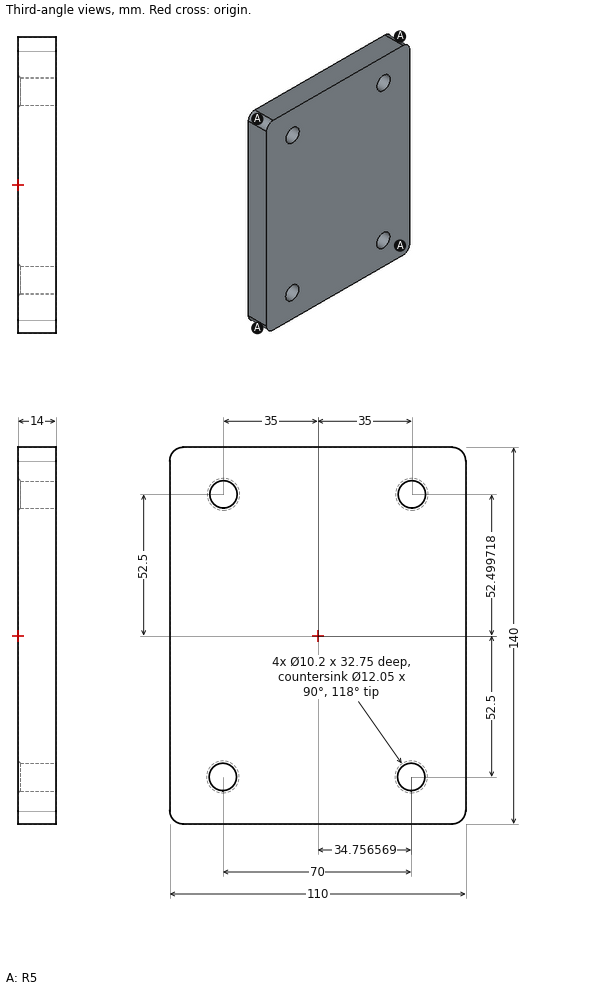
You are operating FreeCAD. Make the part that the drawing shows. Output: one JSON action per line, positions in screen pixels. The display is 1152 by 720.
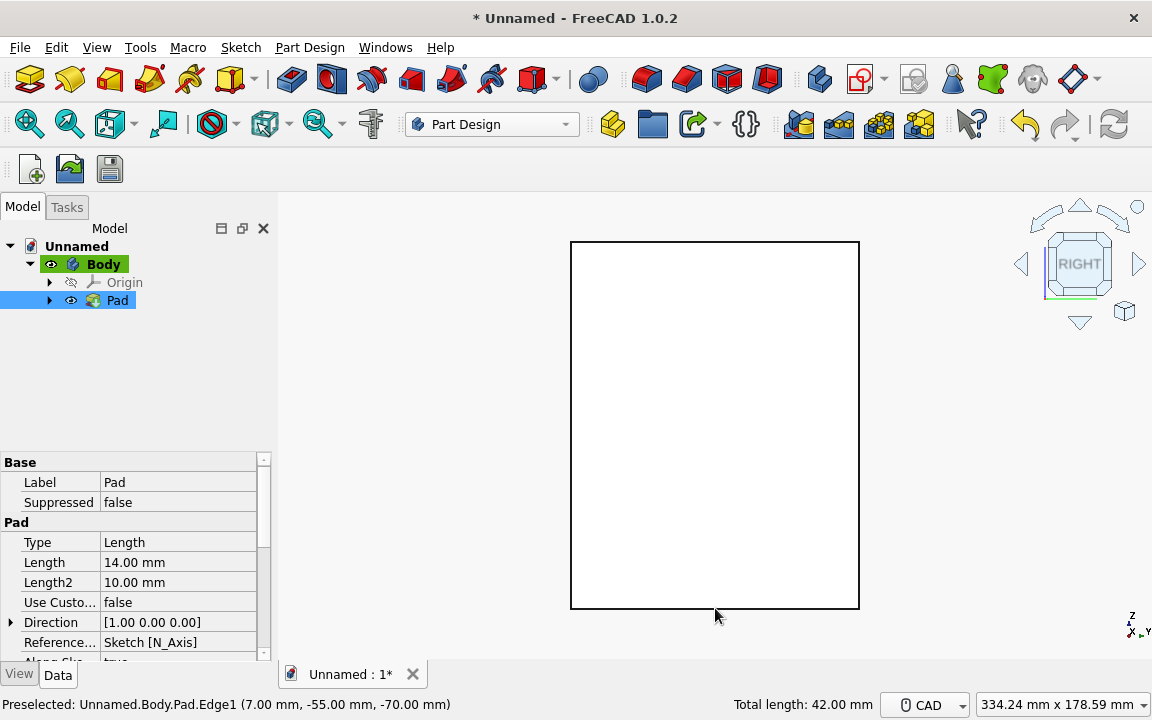
{"action": "key", "text": "5"}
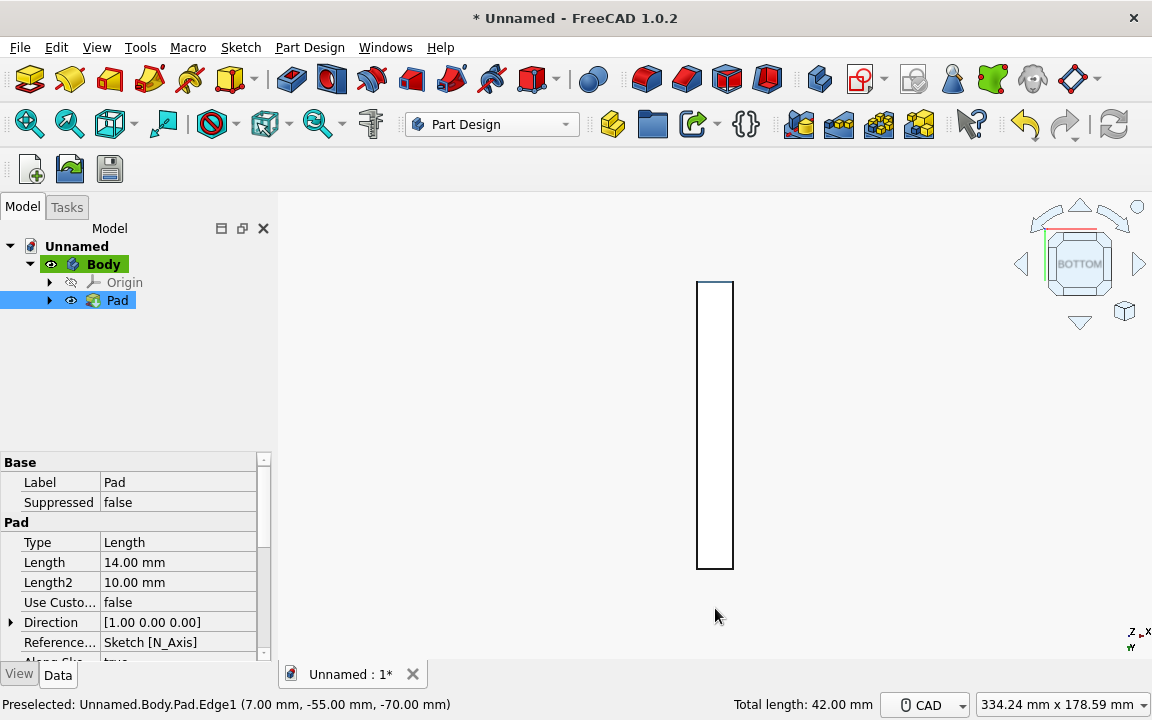
{"action": "left_click", "coordinate": [715, 568], "text": "ctrl"}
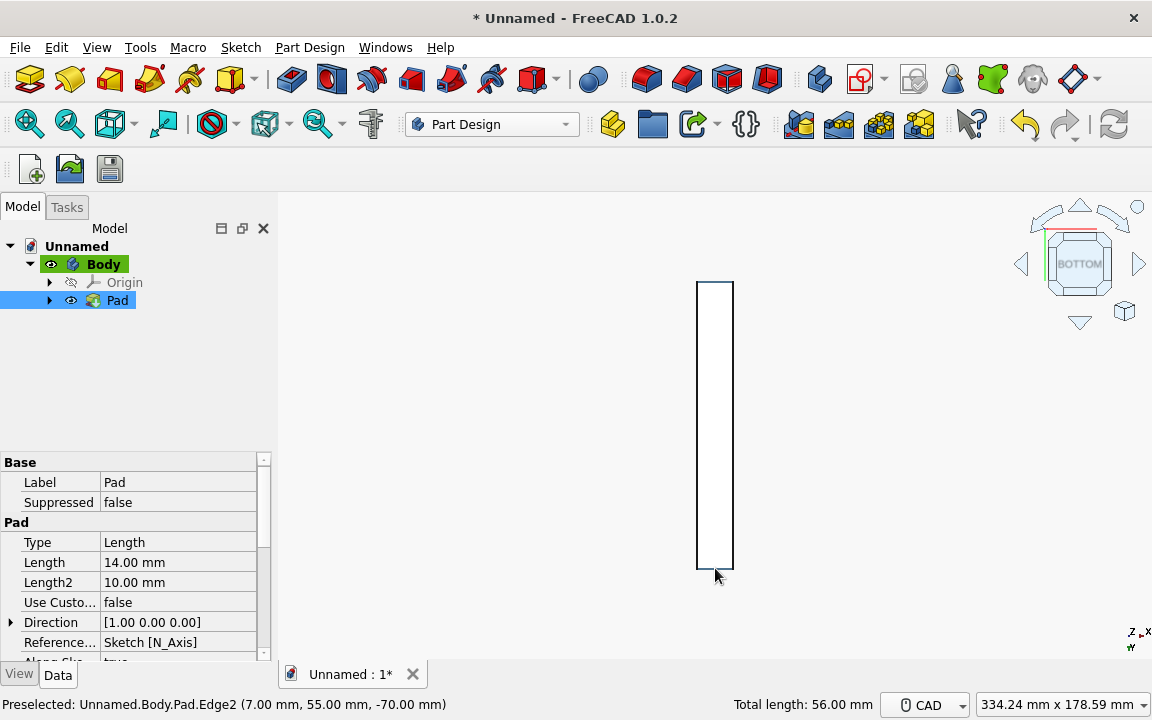
{"action": "left_click", "coordinate": [648, 80]}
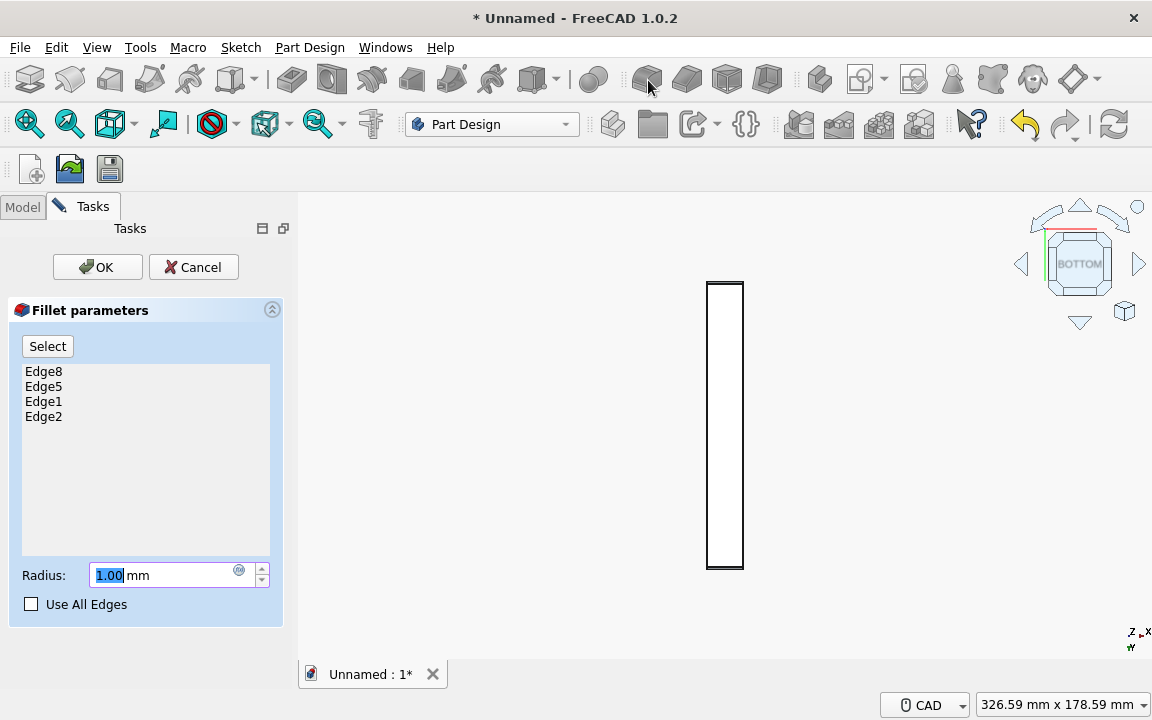
{"action": "type", "text": "5"}
{"action": "key", "text": "Tab"}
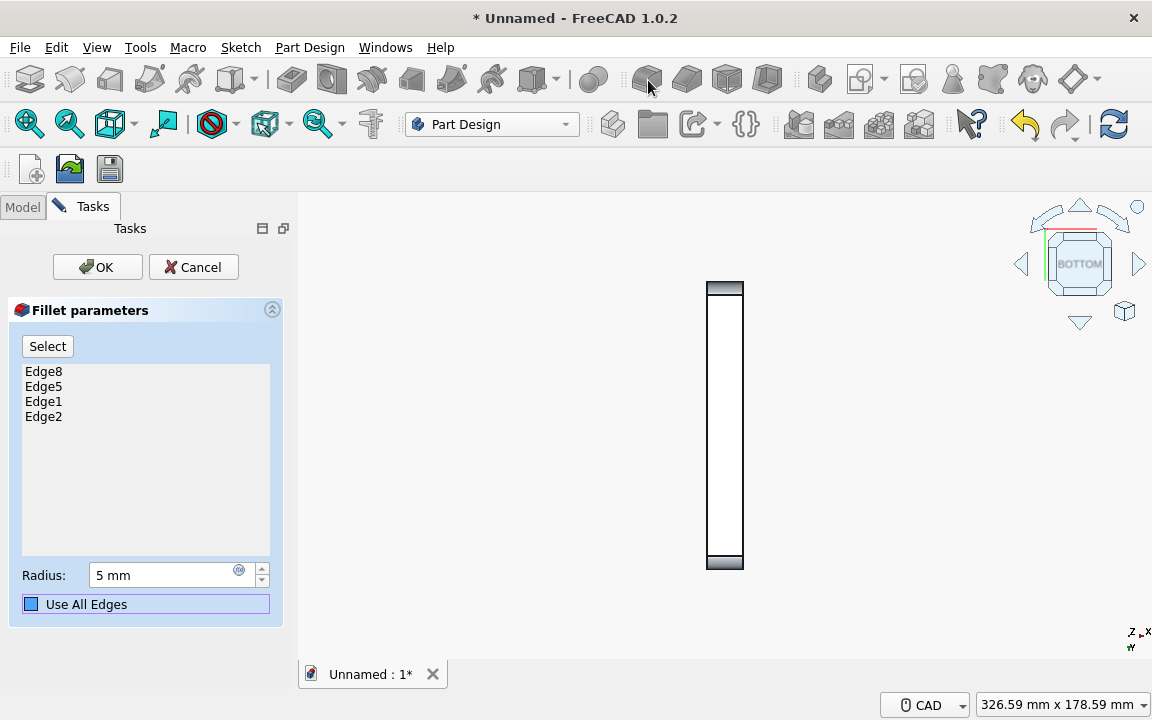
{"action": "left_click", "coordinate": [98, 267]}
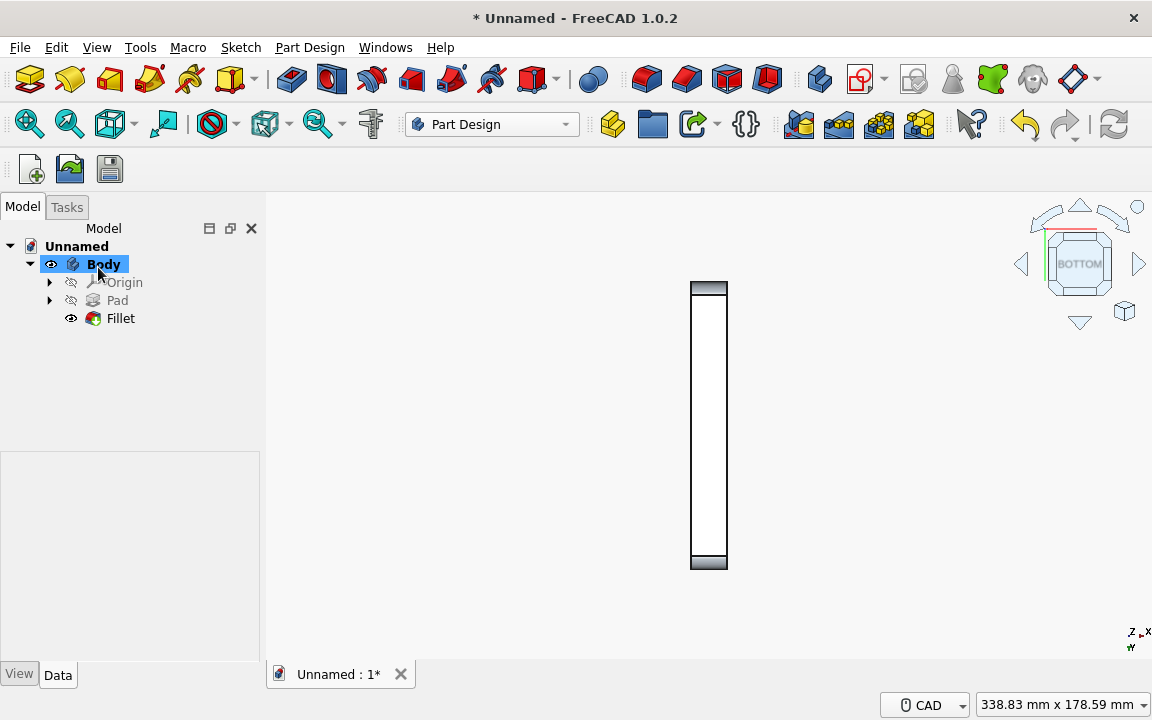
{"action": "key", "text": "6"}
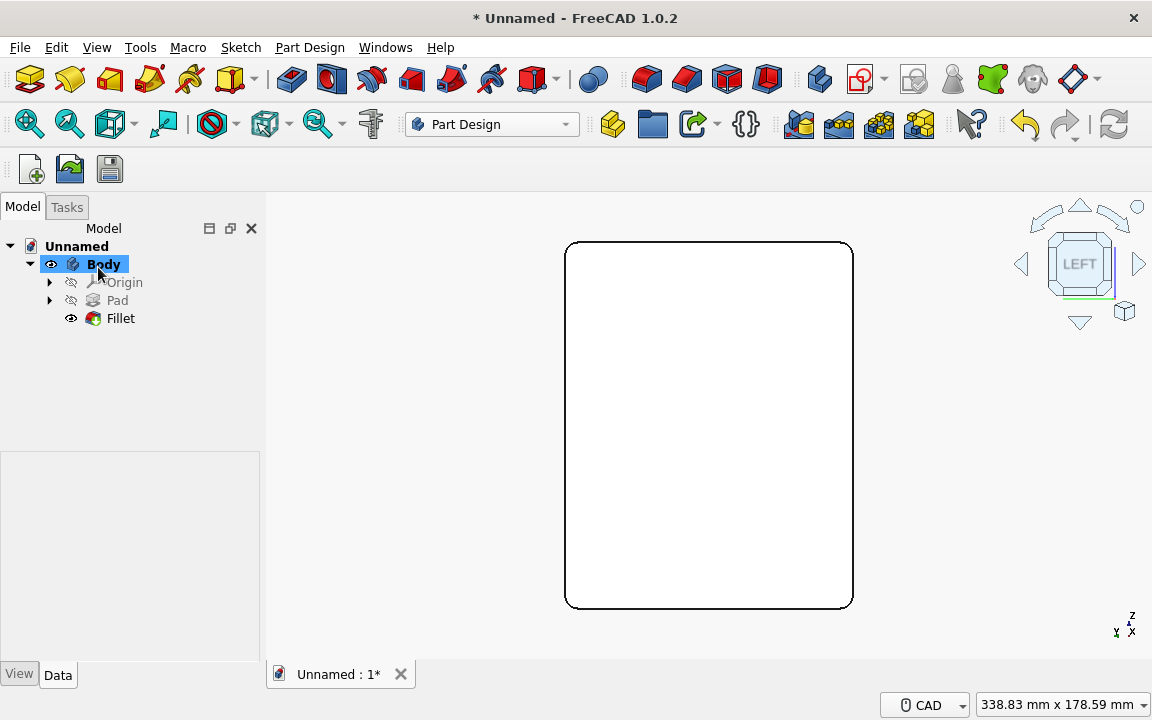
{"action": "left_click", "coordinate": [709, 424]}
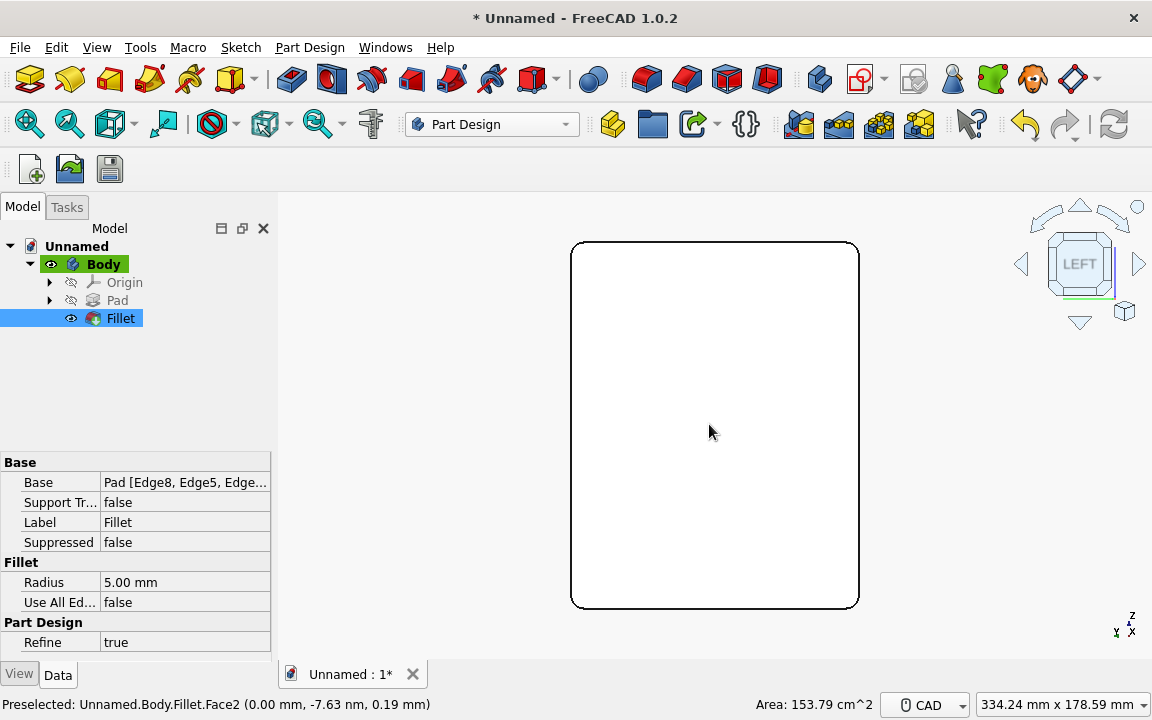
{"action": "left_click", "coordinate": [860, 80]}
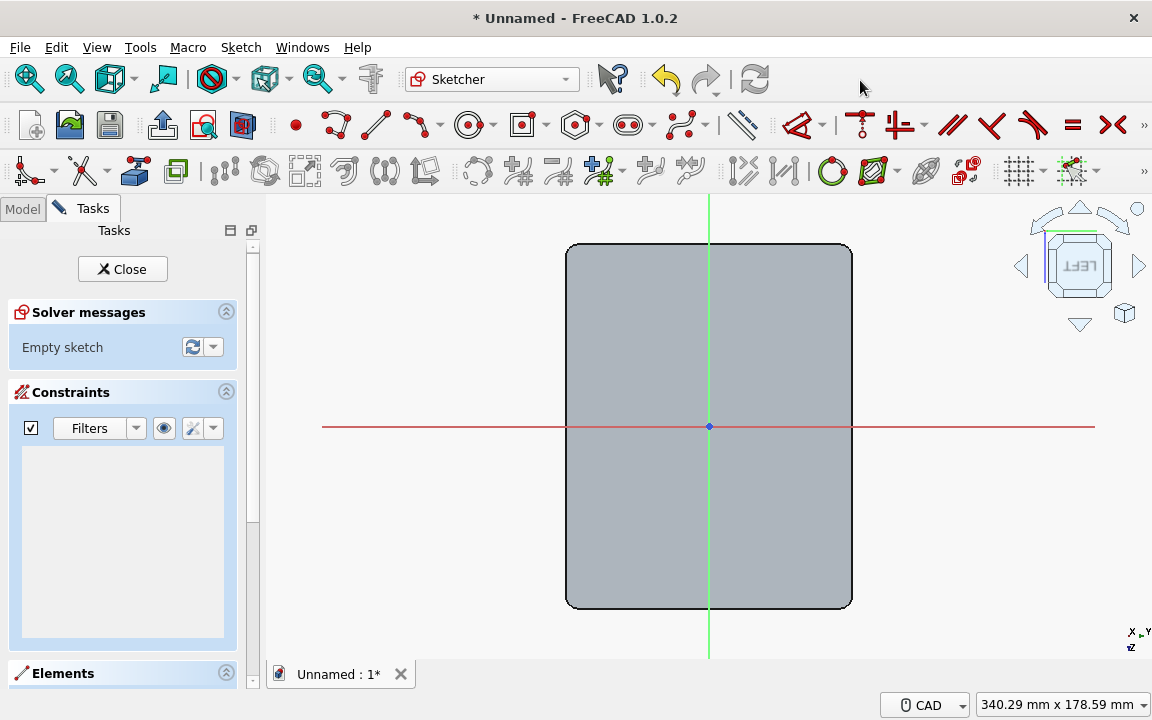
{"action": "left_click", "coordinate": [470, 126]}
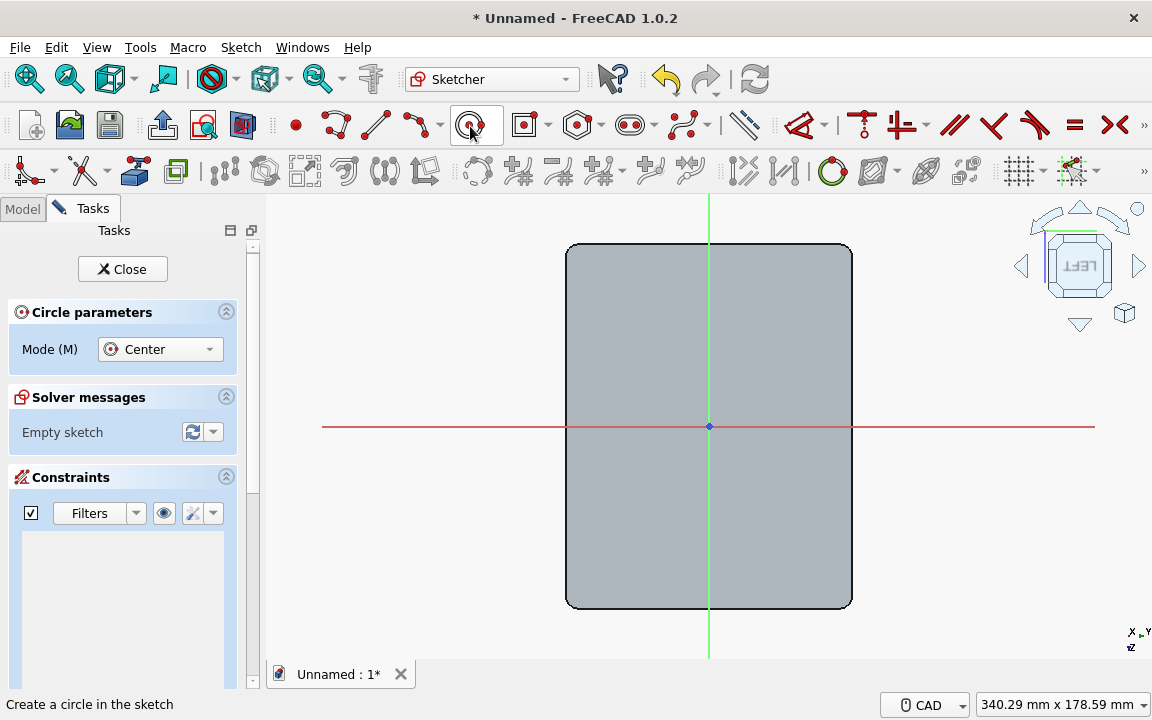
{"action": "scroll", "coordinate": [799, 290], "scroll_direction": "up", "scroll_amount": 3}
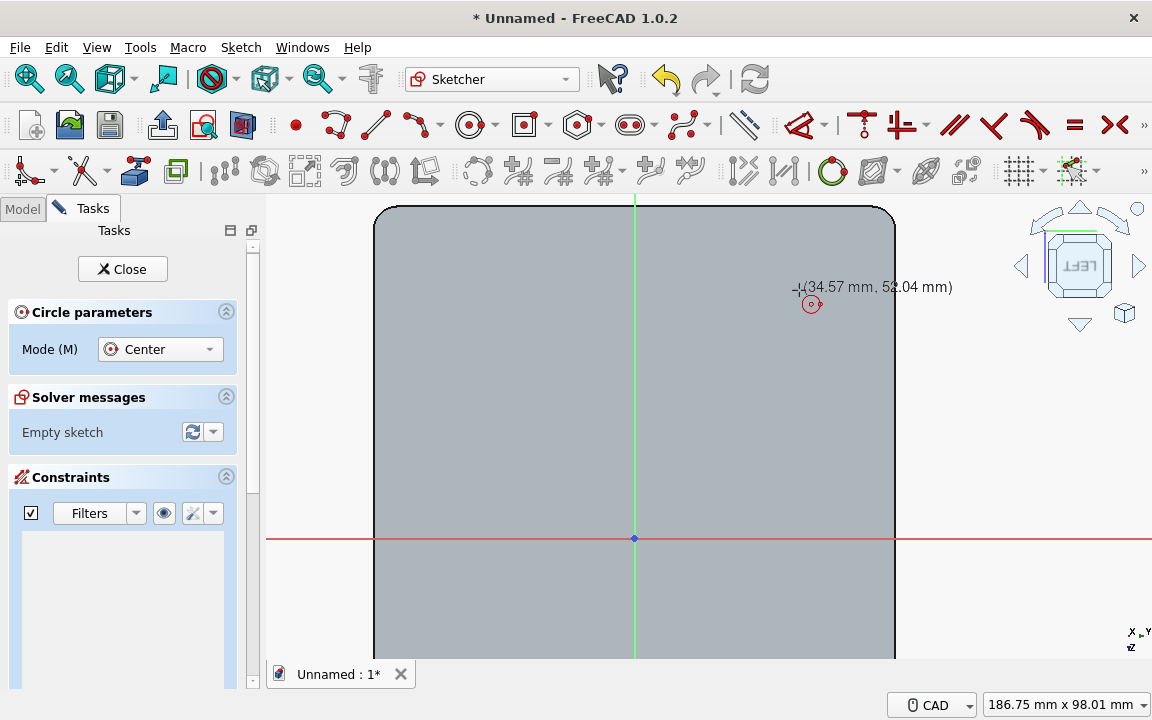
{"action": "left_click", "coordinate": [799, 289]}
{"action": "left_click", "coordinate": [817, 272]}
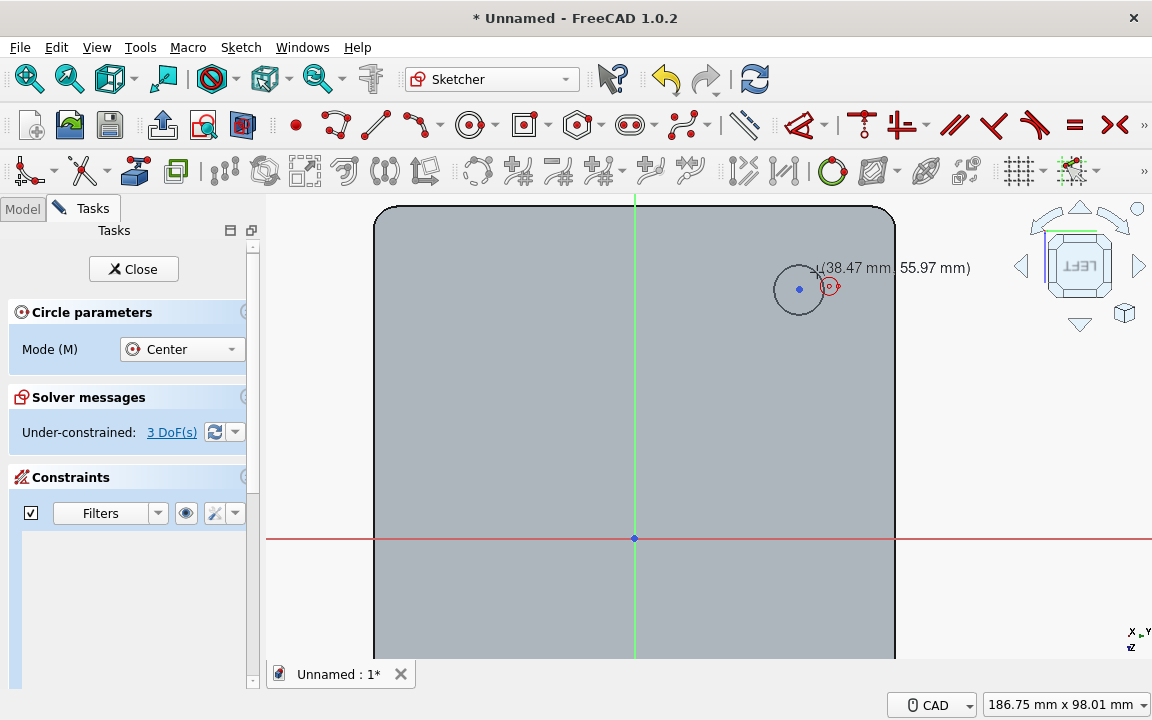
{"action": "scroll", "coordinate": [648, 290], "scroll_direction": "down", "scroll_amount": 3}